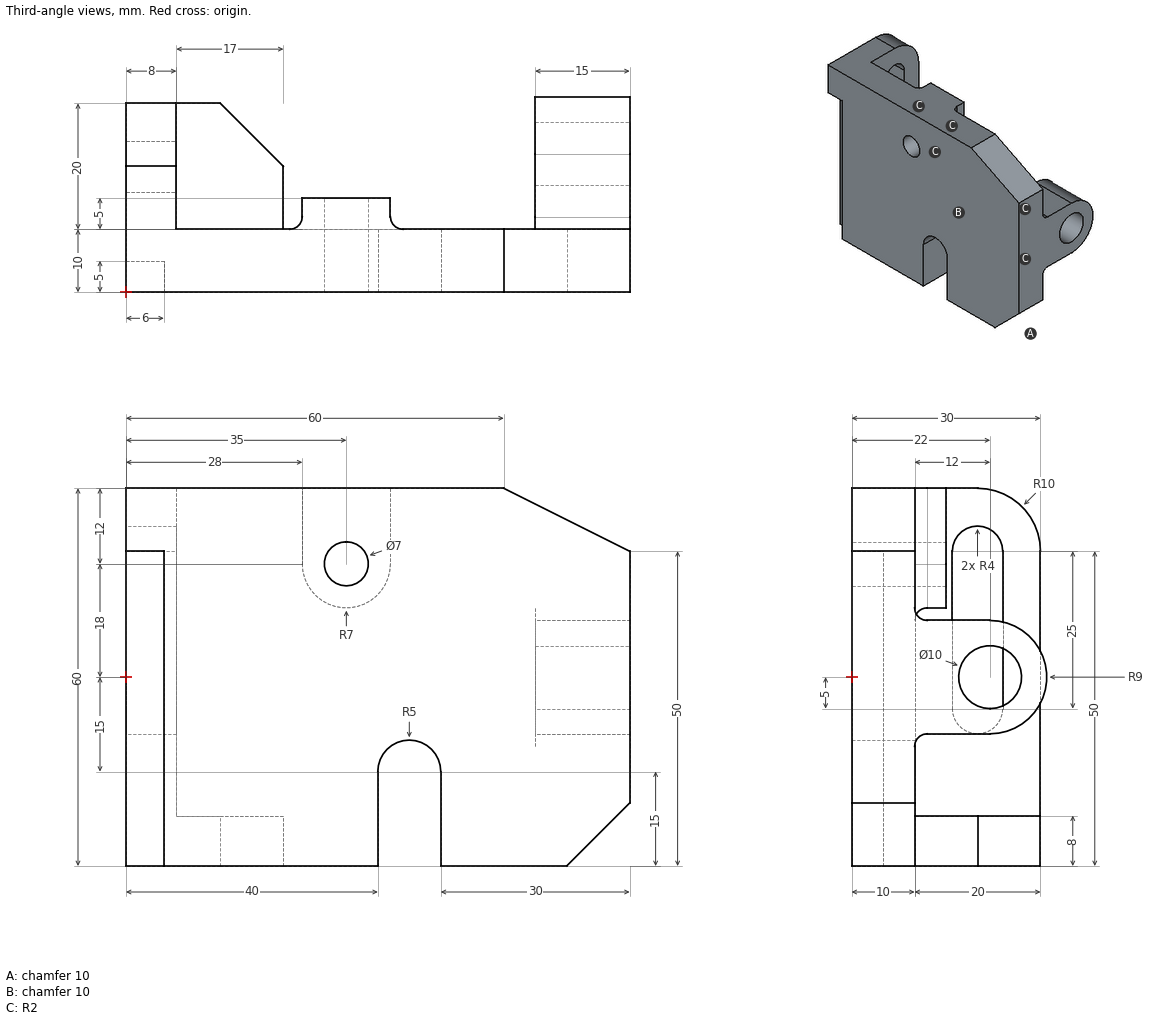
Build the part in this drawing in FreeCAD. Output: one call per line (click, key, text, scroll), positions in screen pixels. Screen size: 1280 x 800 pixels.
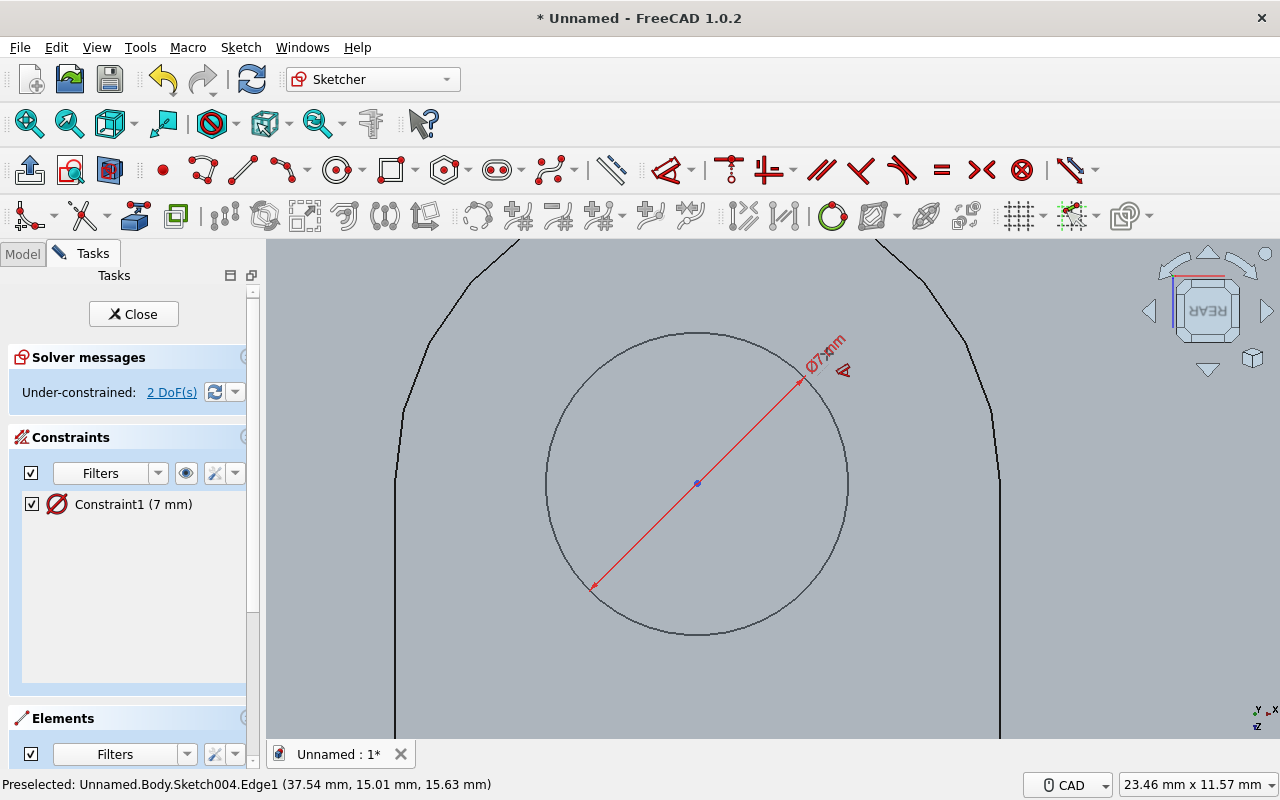
click(697, 484)
click(495, 518)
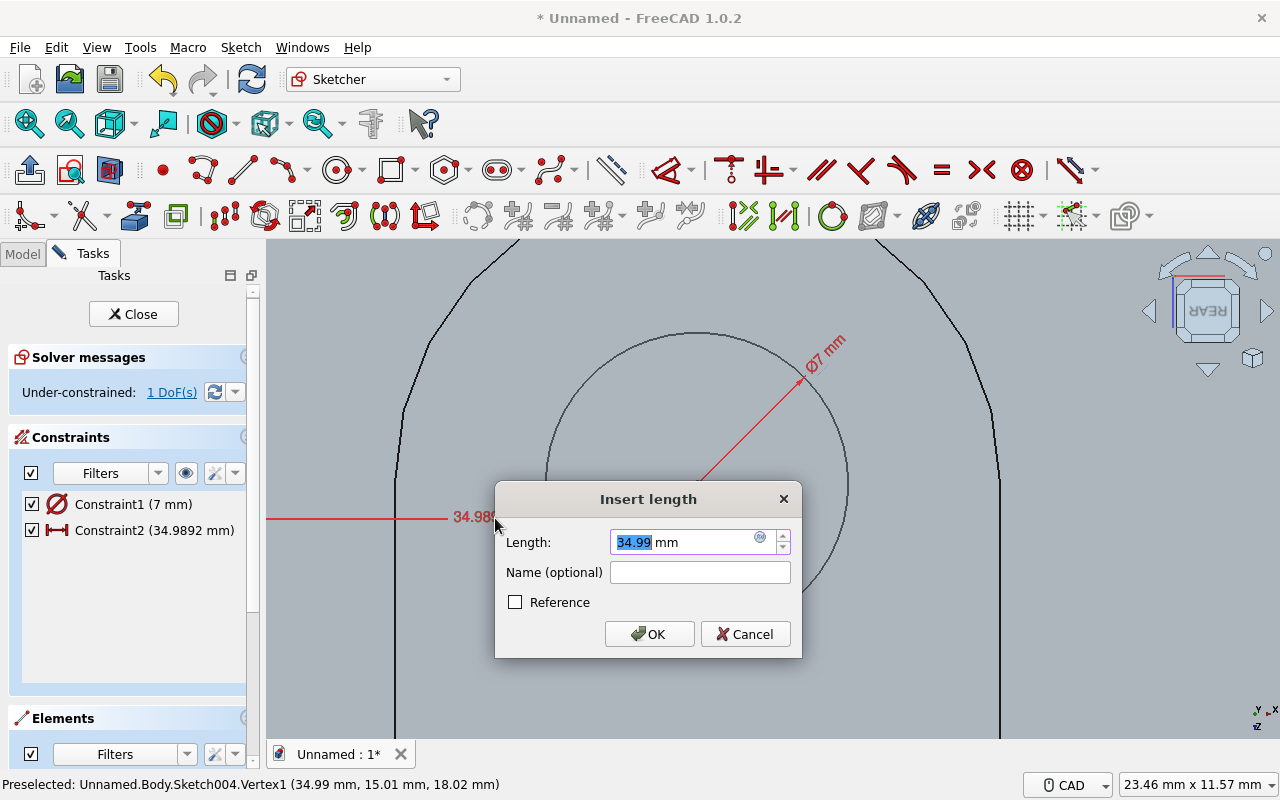
text(35)
key(Return)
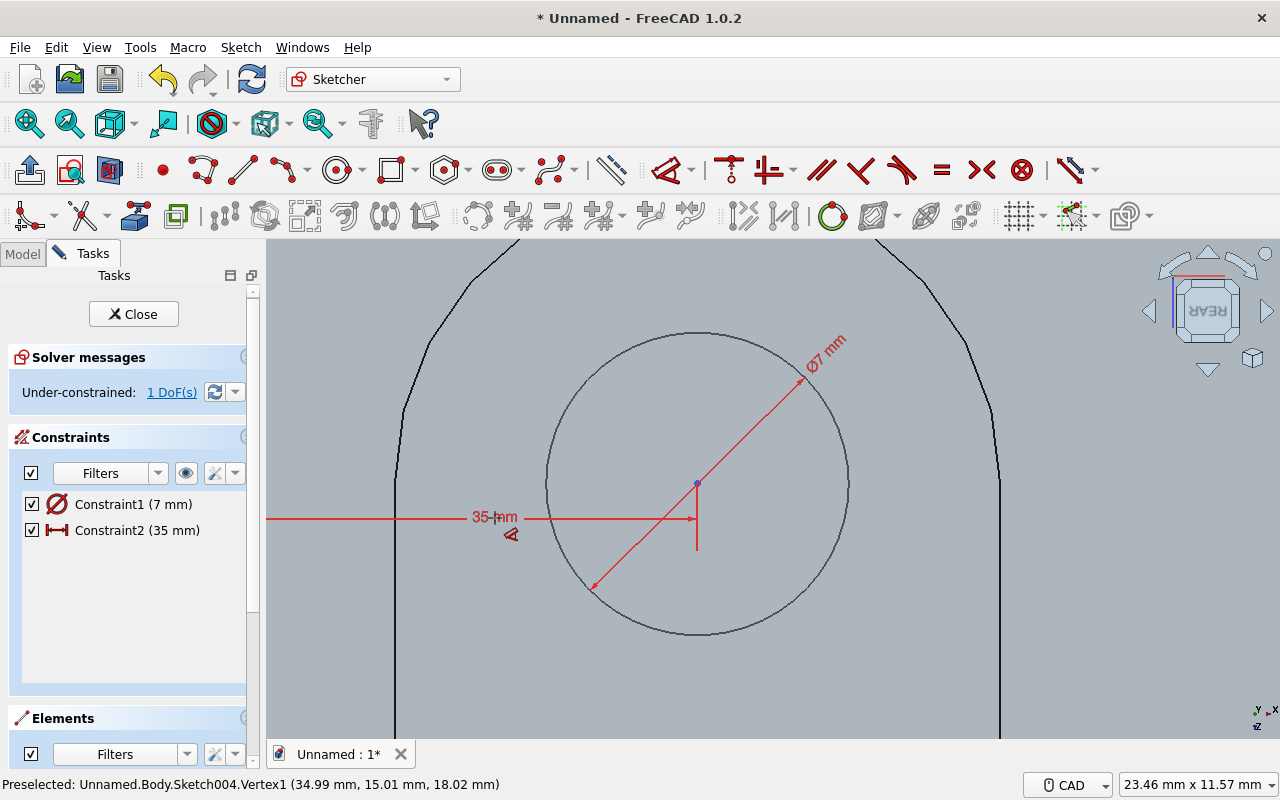
click(697, 484)
click(731, 375)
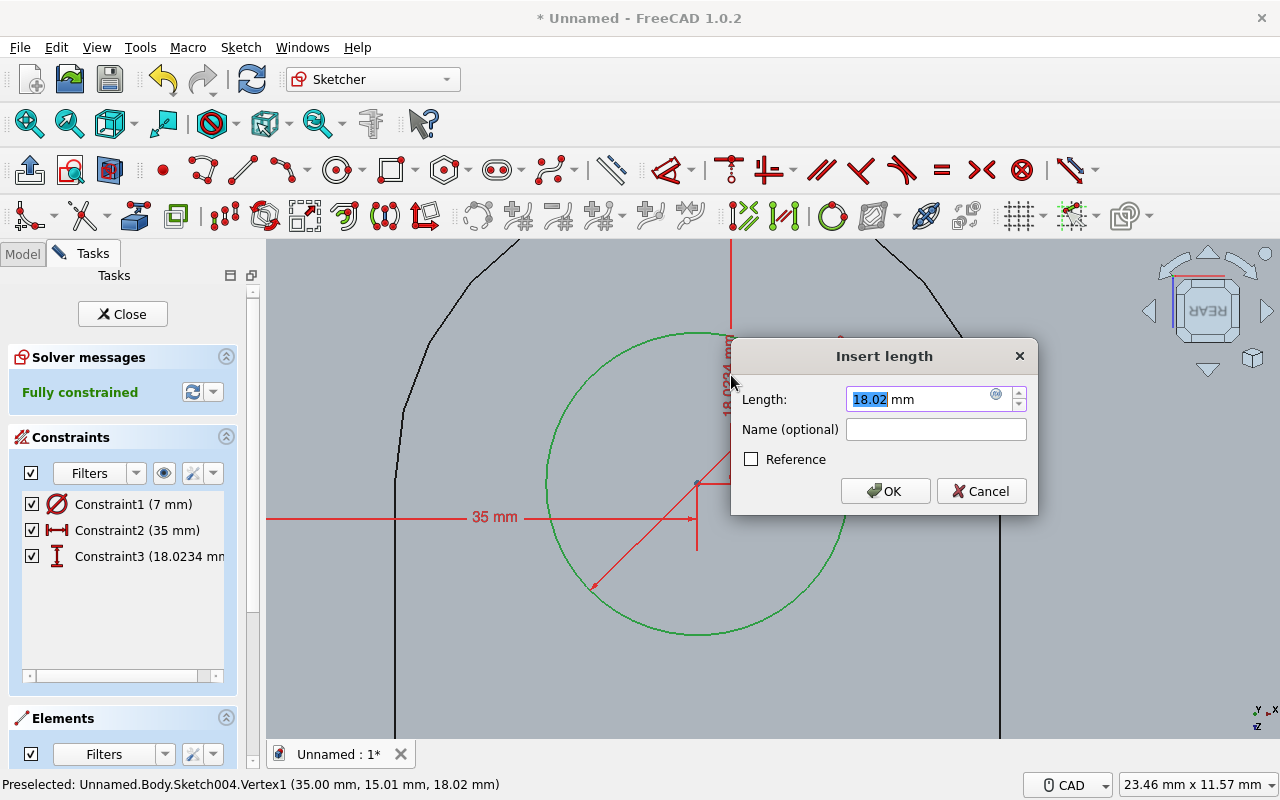
text(18)
key(Return)
key(Escape)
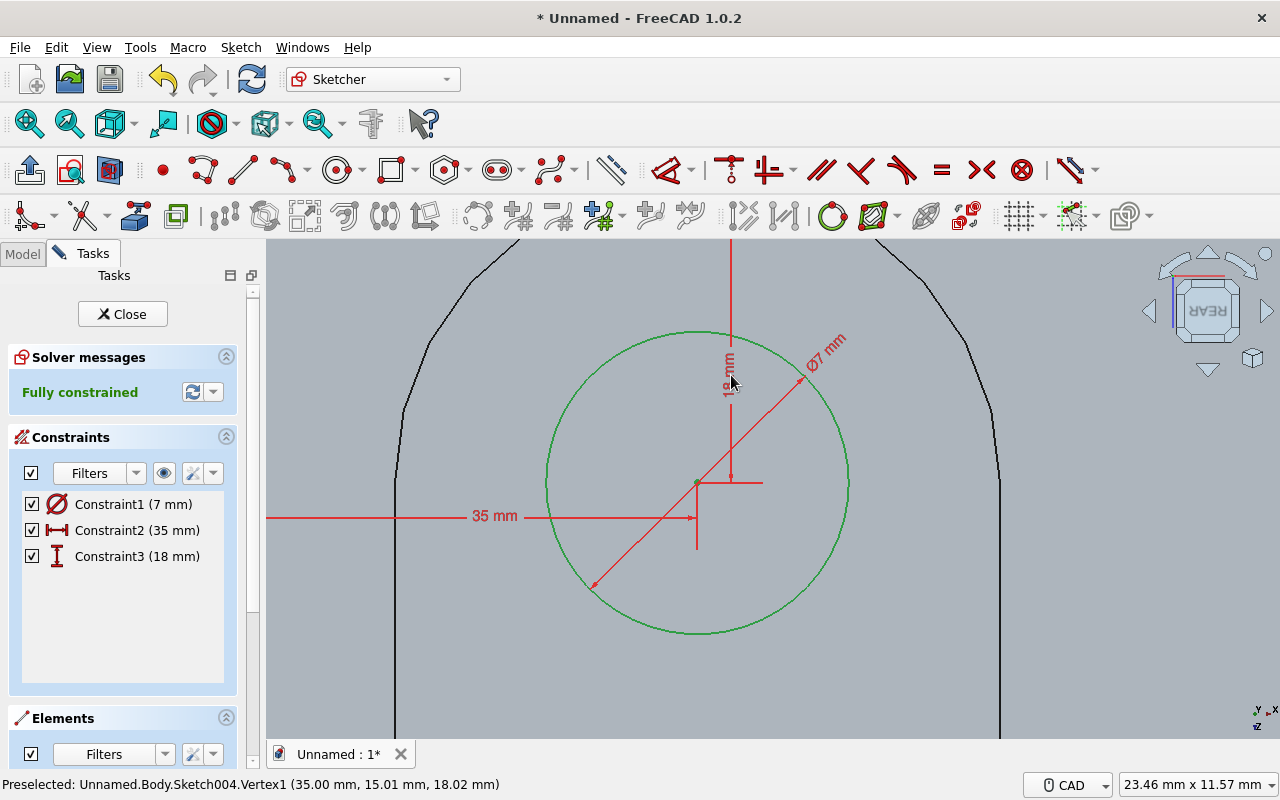
click(123, 314)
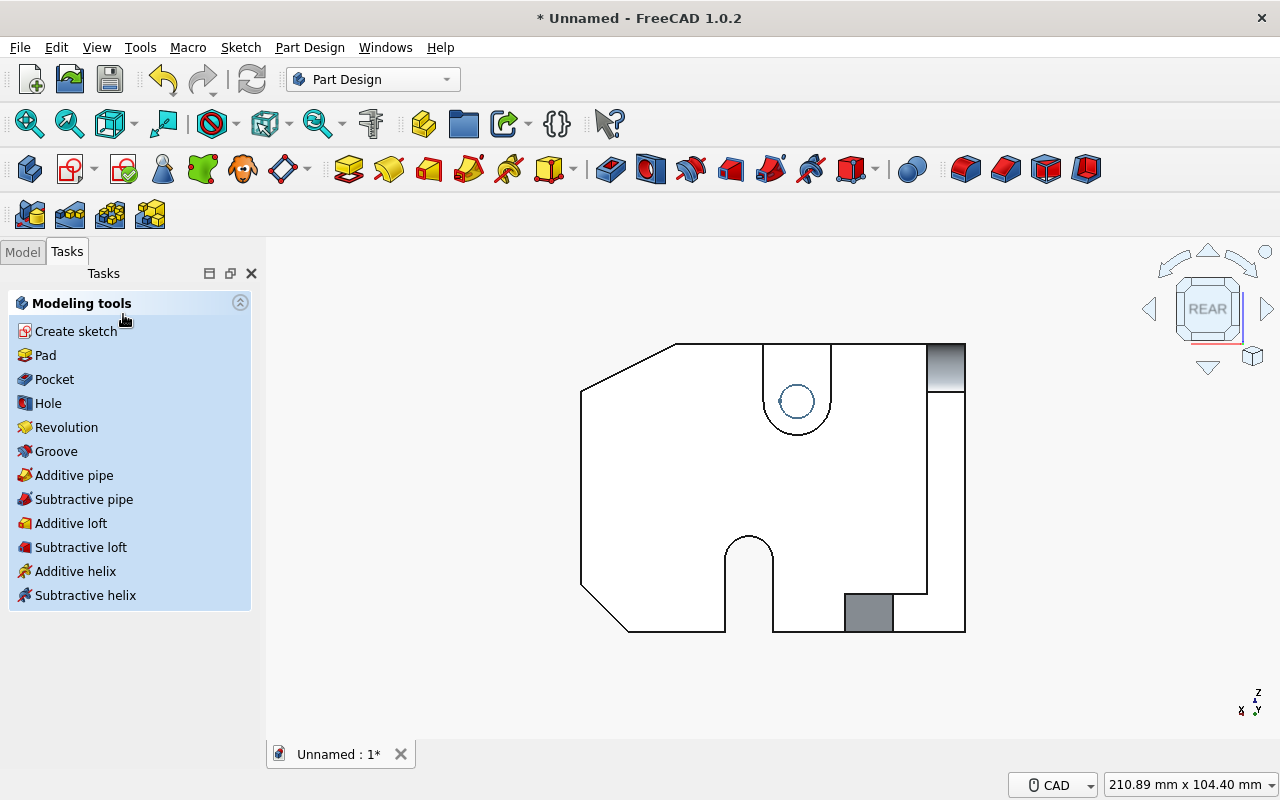
click(612, 170)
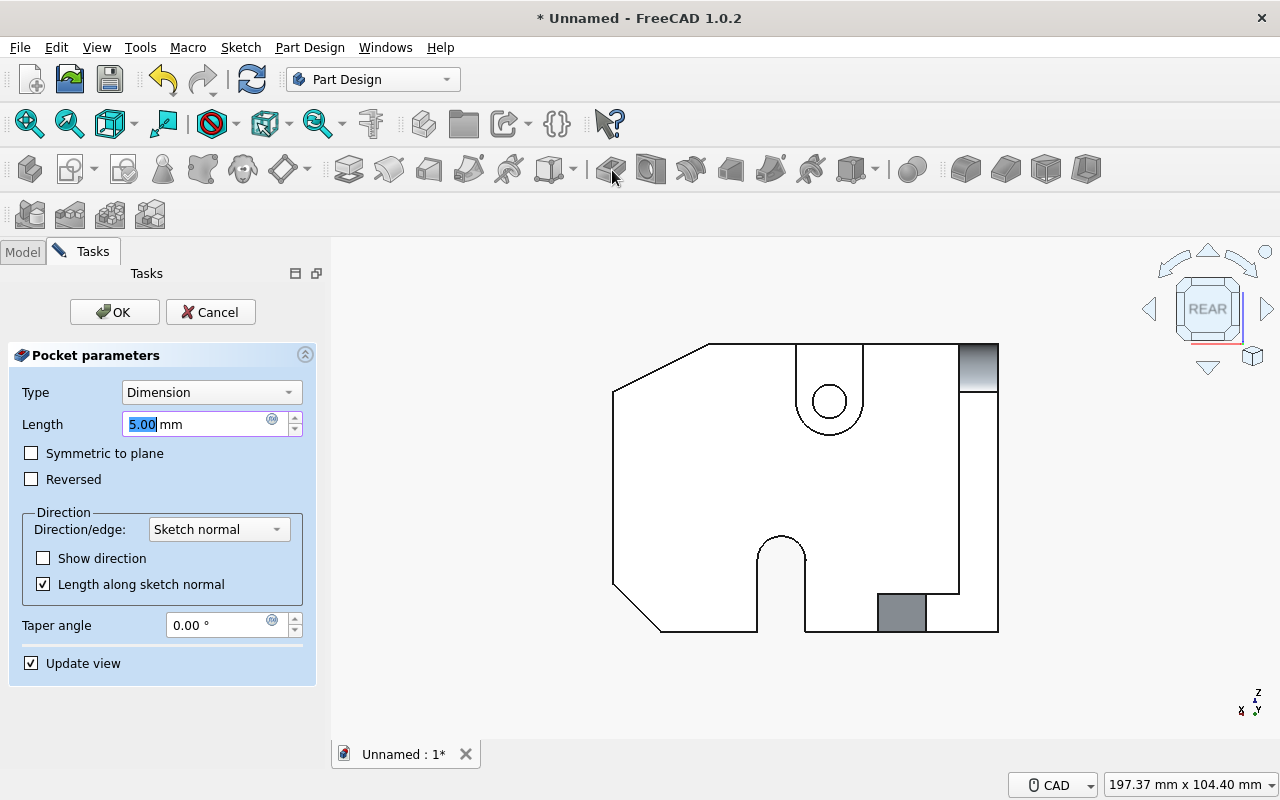
click(212, 392)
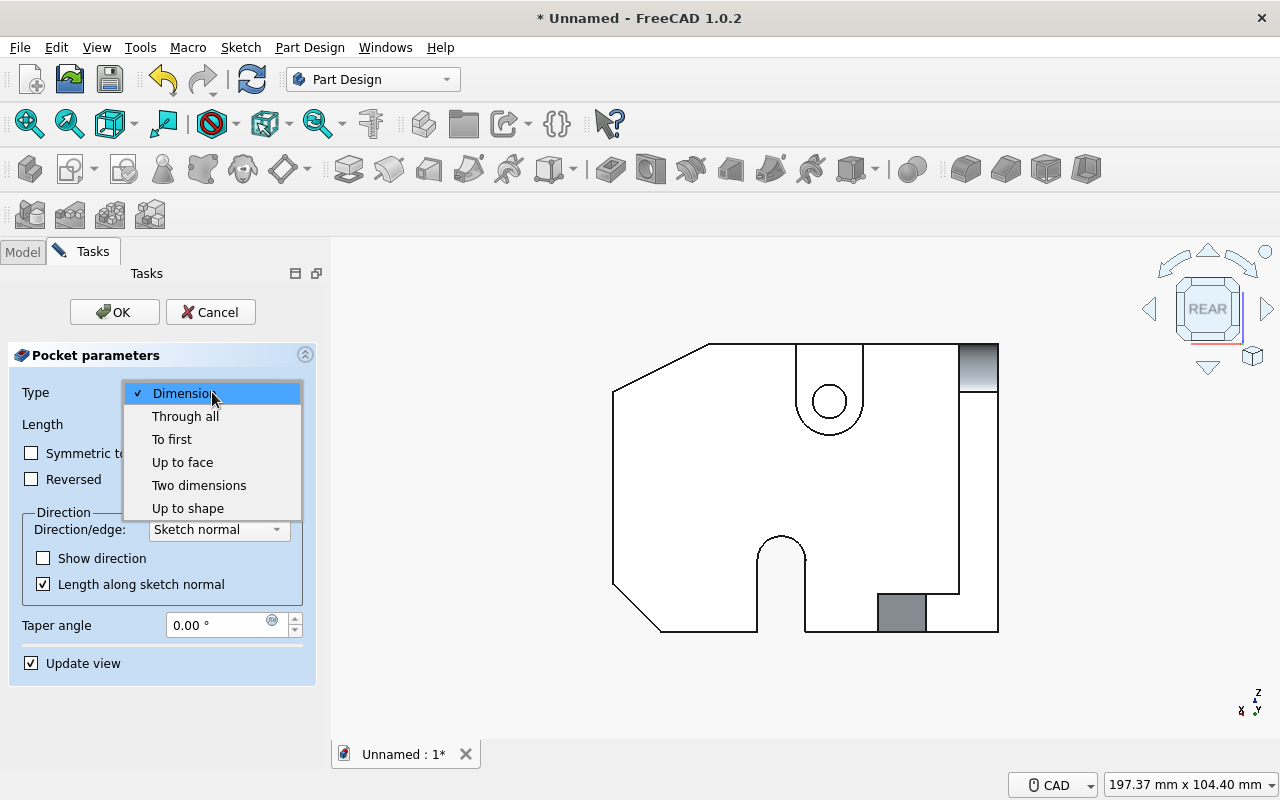
click(212, 416)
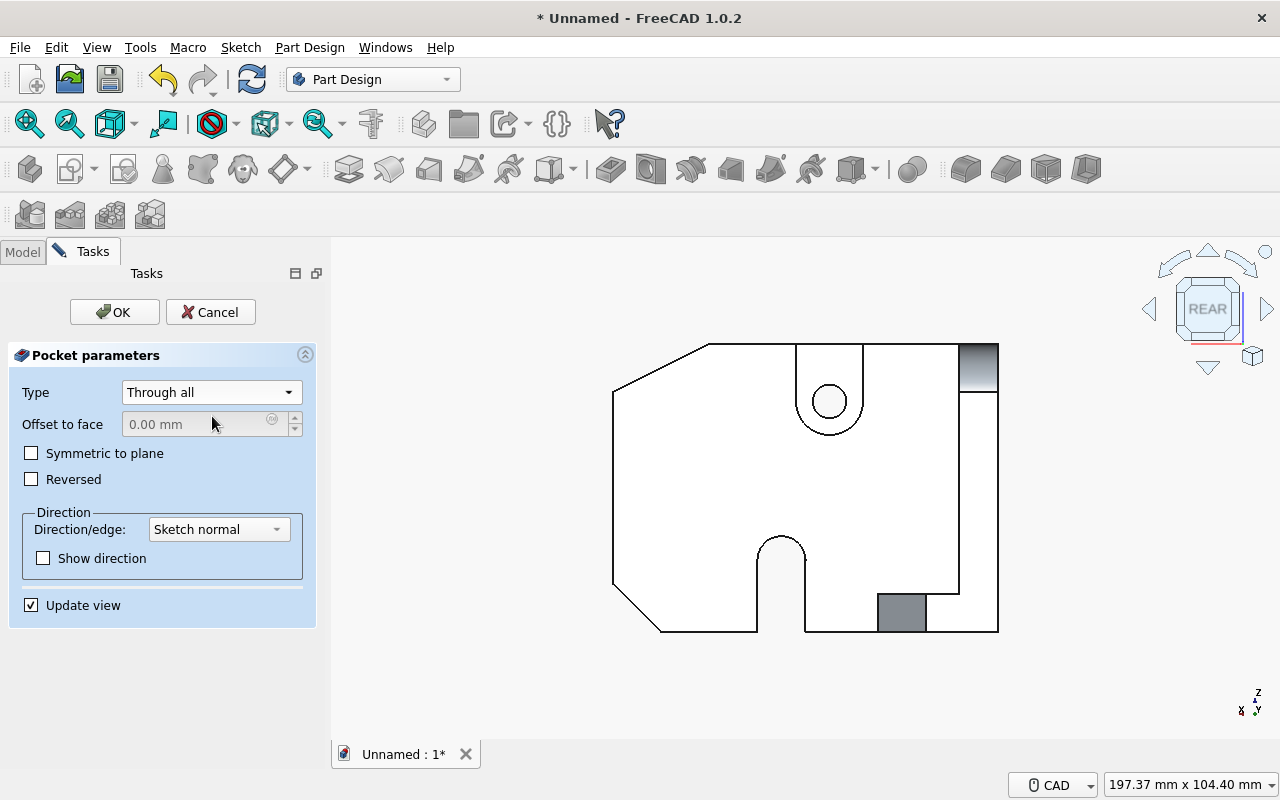
click(115, 312)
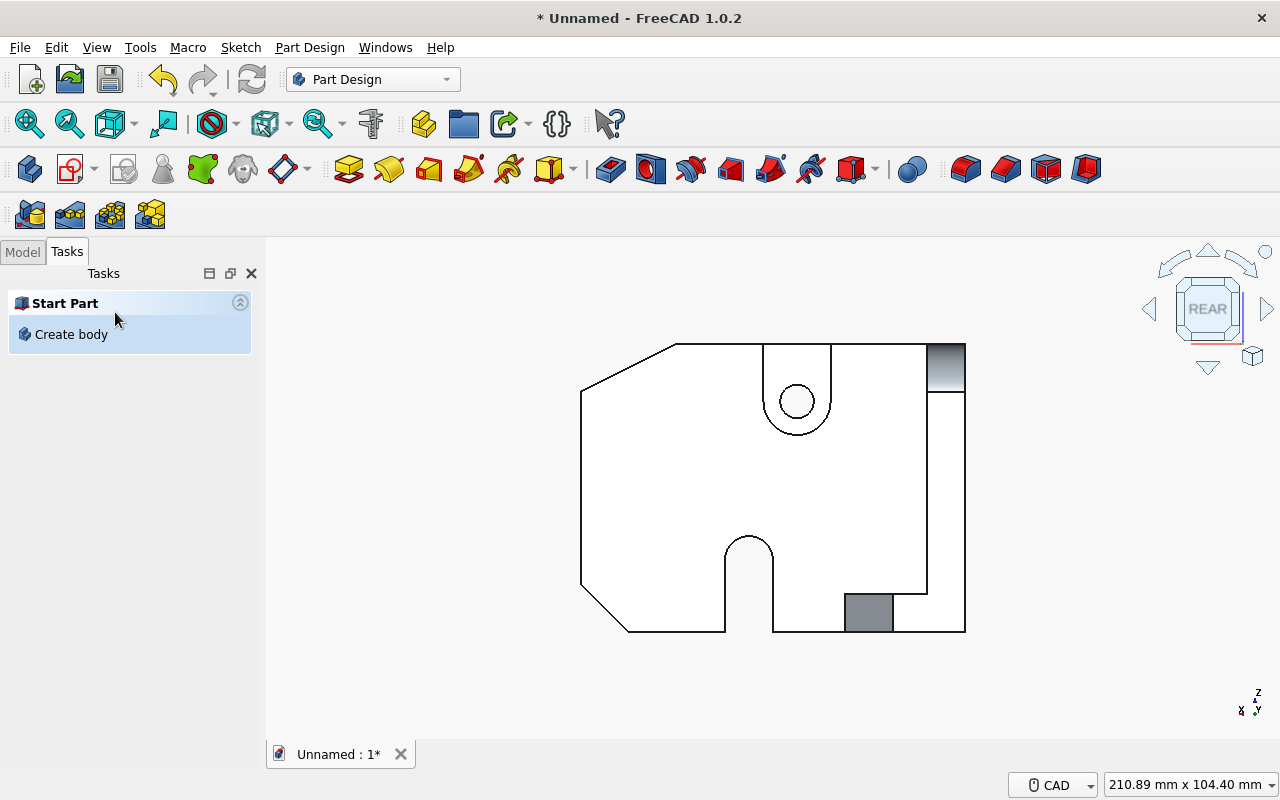
key(0)